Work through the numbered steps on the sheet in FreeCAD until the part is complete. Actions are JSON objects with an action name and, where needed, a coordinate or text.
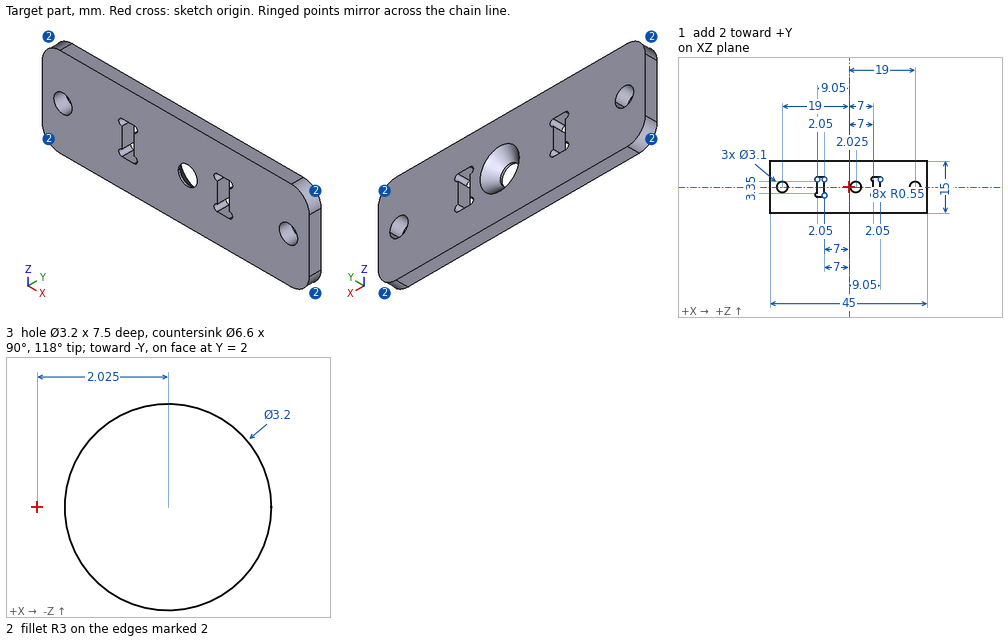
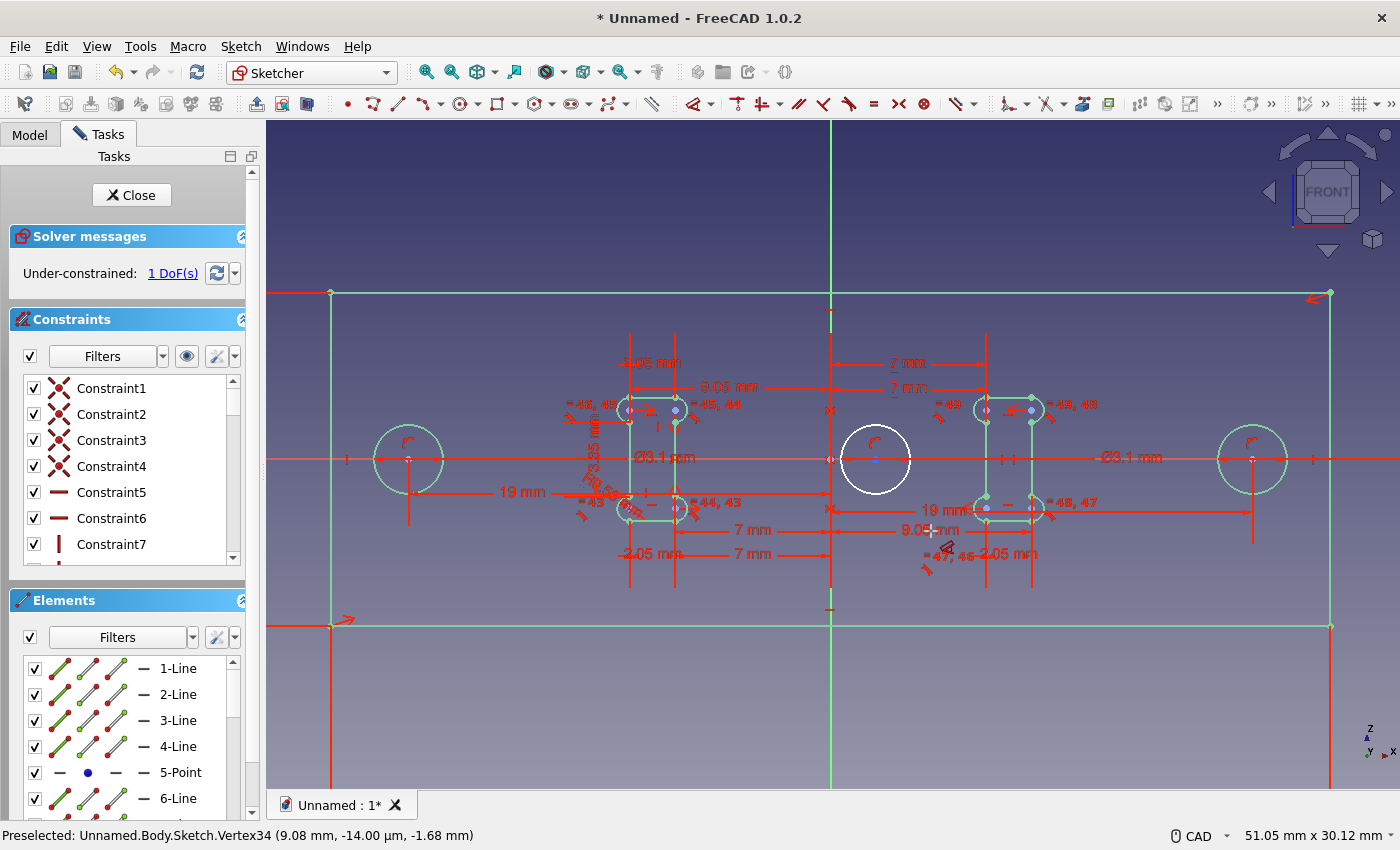
{"action": "left_click", "coordinate": [876, 459]}
{"action": "left_click", "coordinate": [853, 517]}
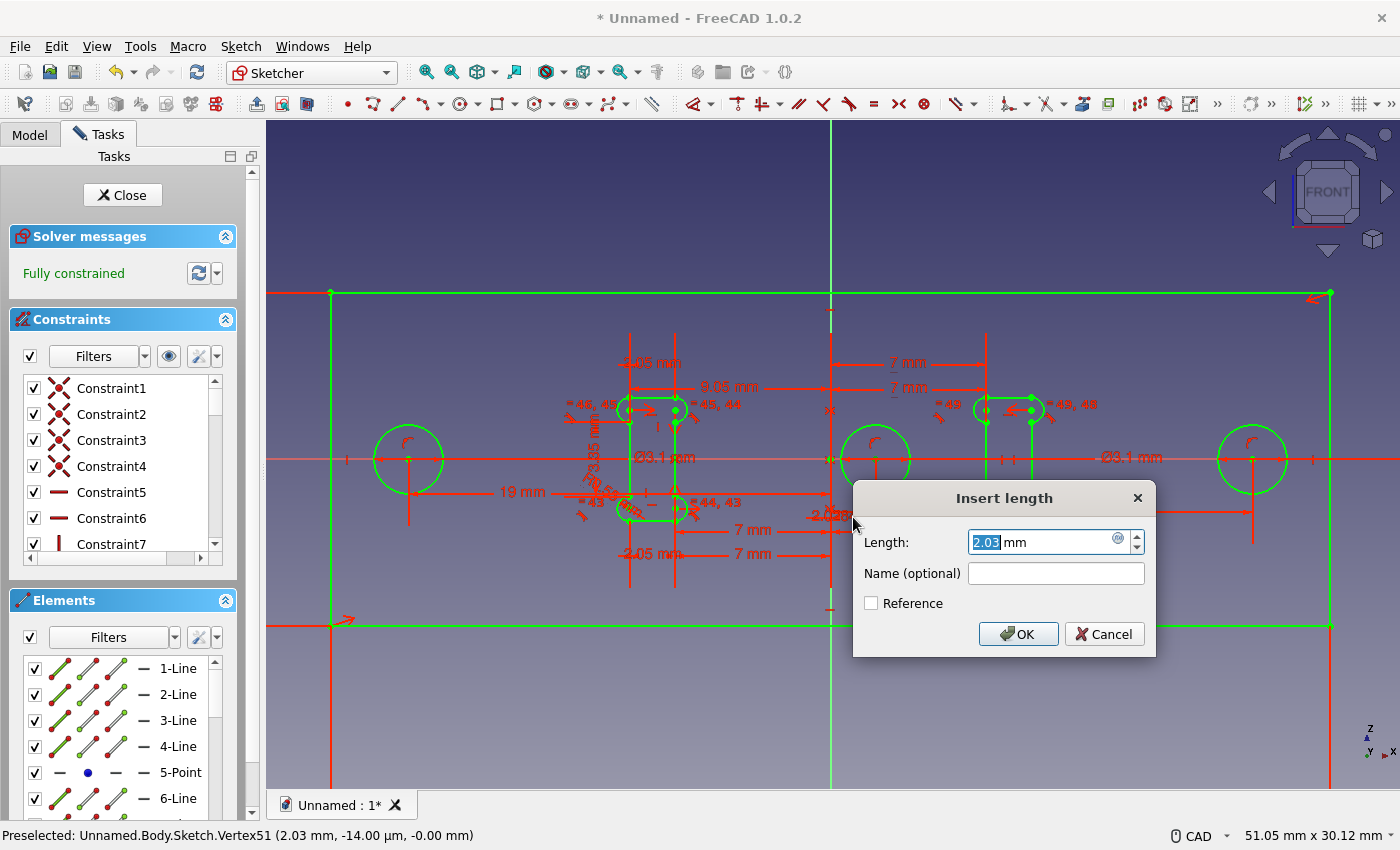
{"action": "type", "text": "2.025"}
{"action": "key", "text": "Return"}
{"action": "key", "text": "Escape"}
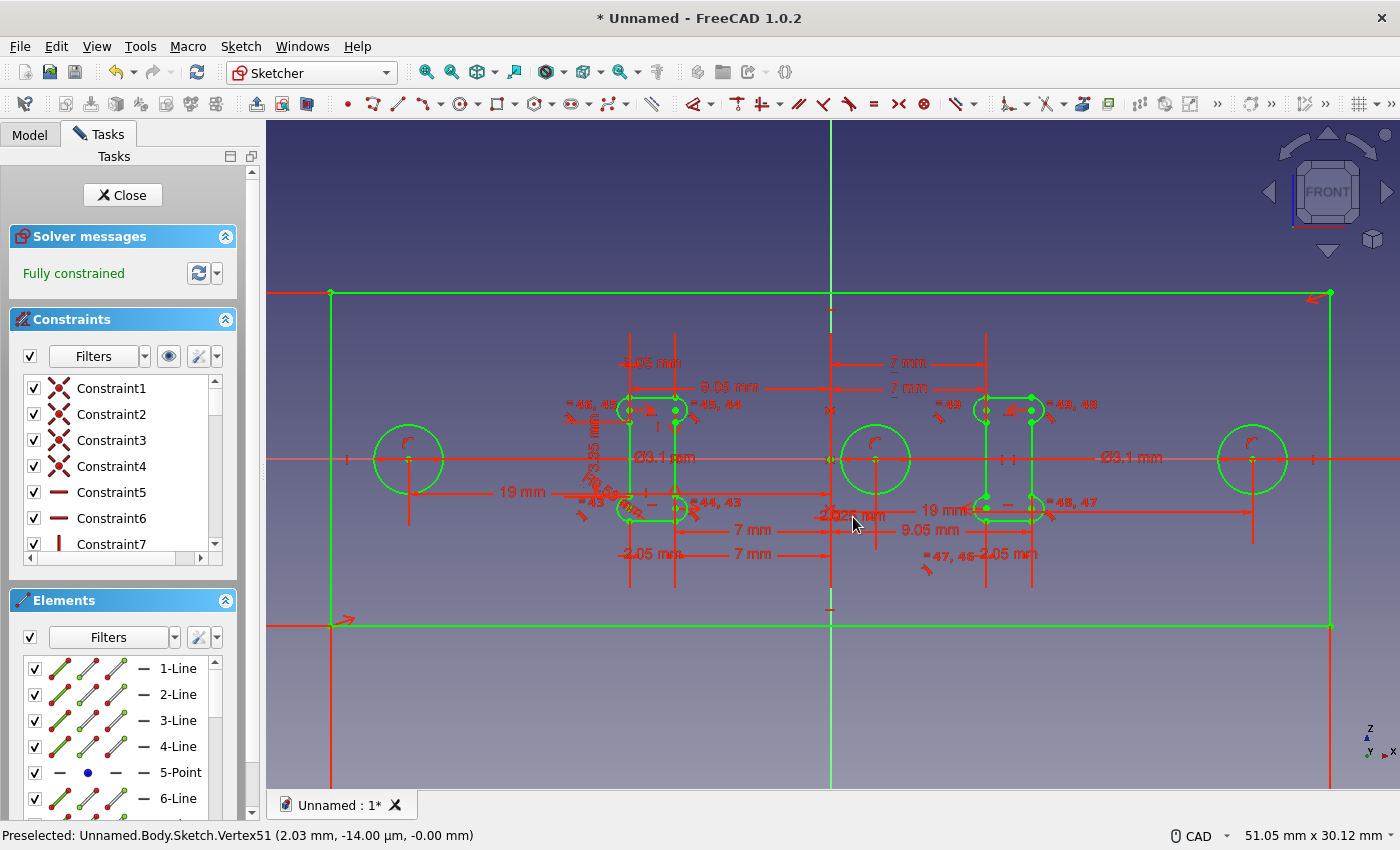
{"action": "left_click", "coordinate": [123, 195]}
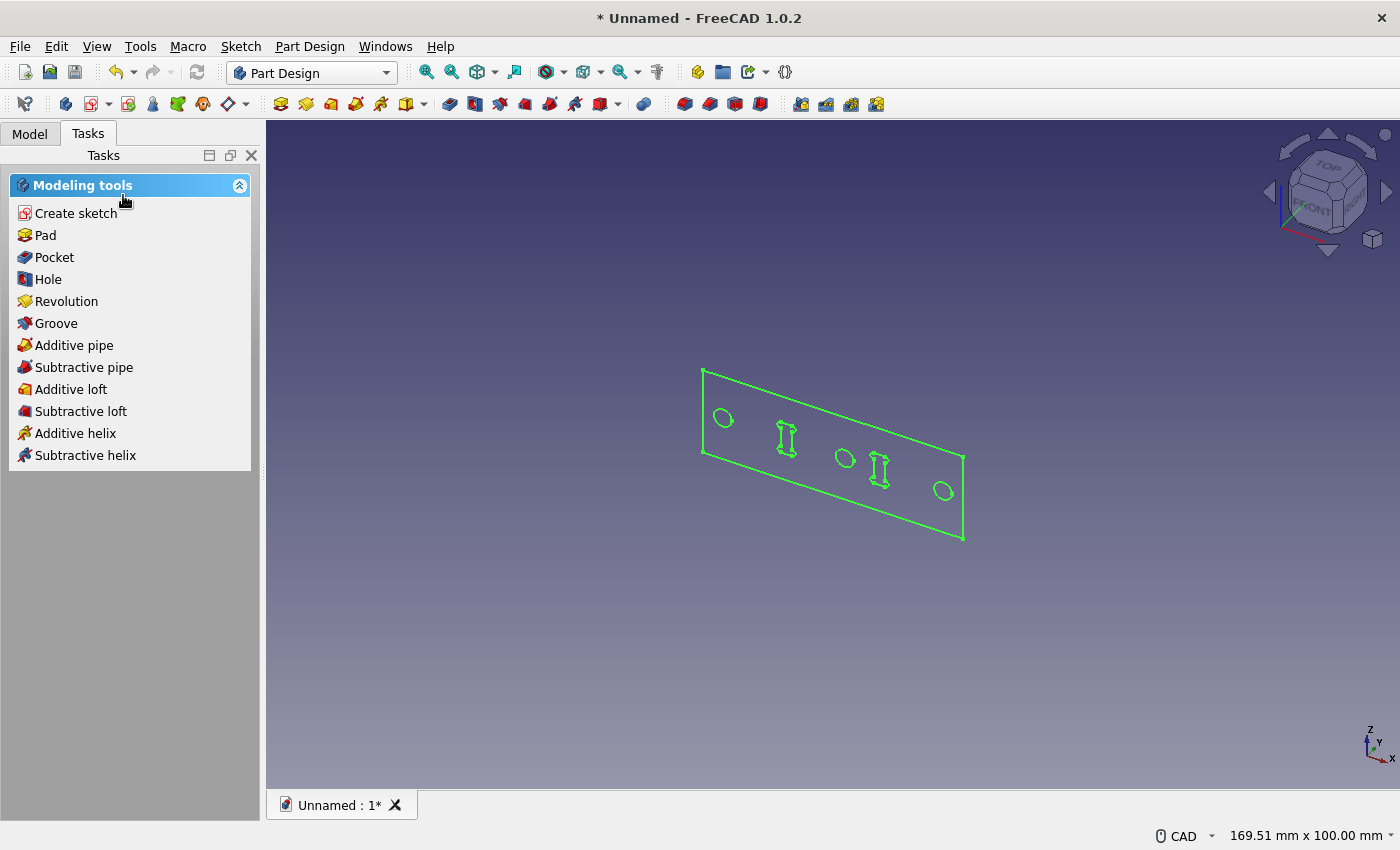
{"action": "left_click", "coordinate": [281, 104]}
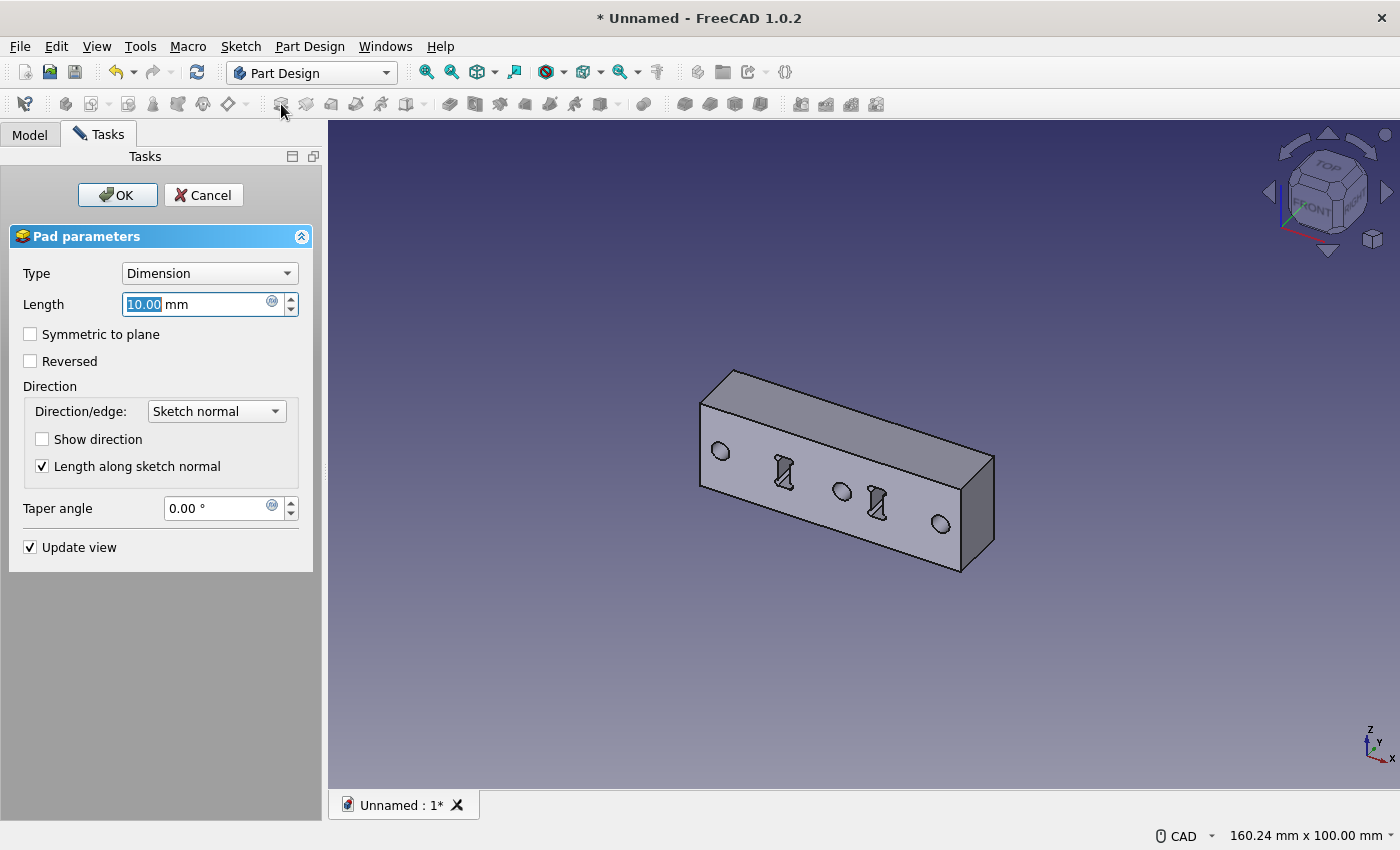
{"action": "type", "text": "2"}
{"action": "key", "text": "Tab"}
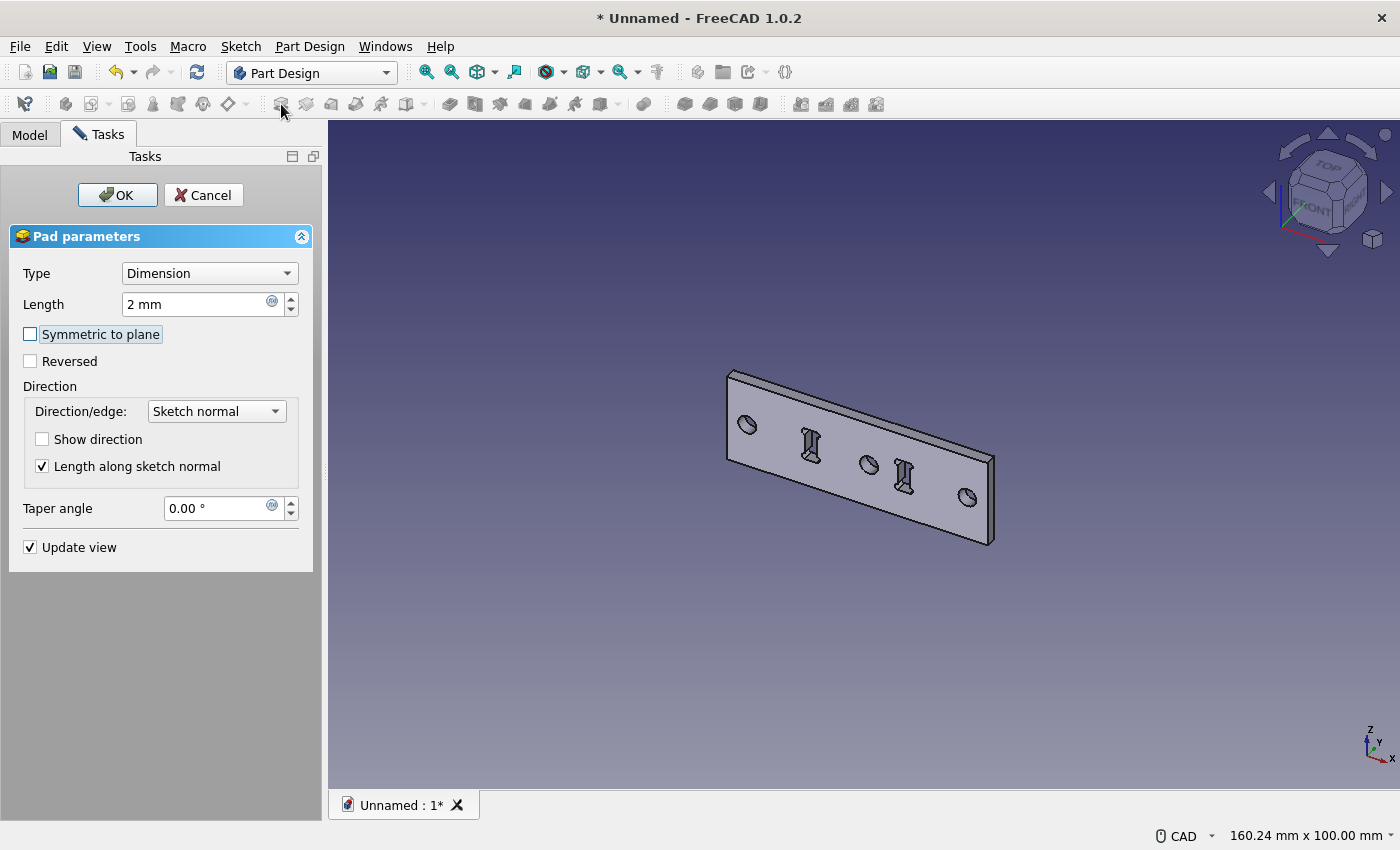
{"action": "left_click", "coordinate": [31, 361]}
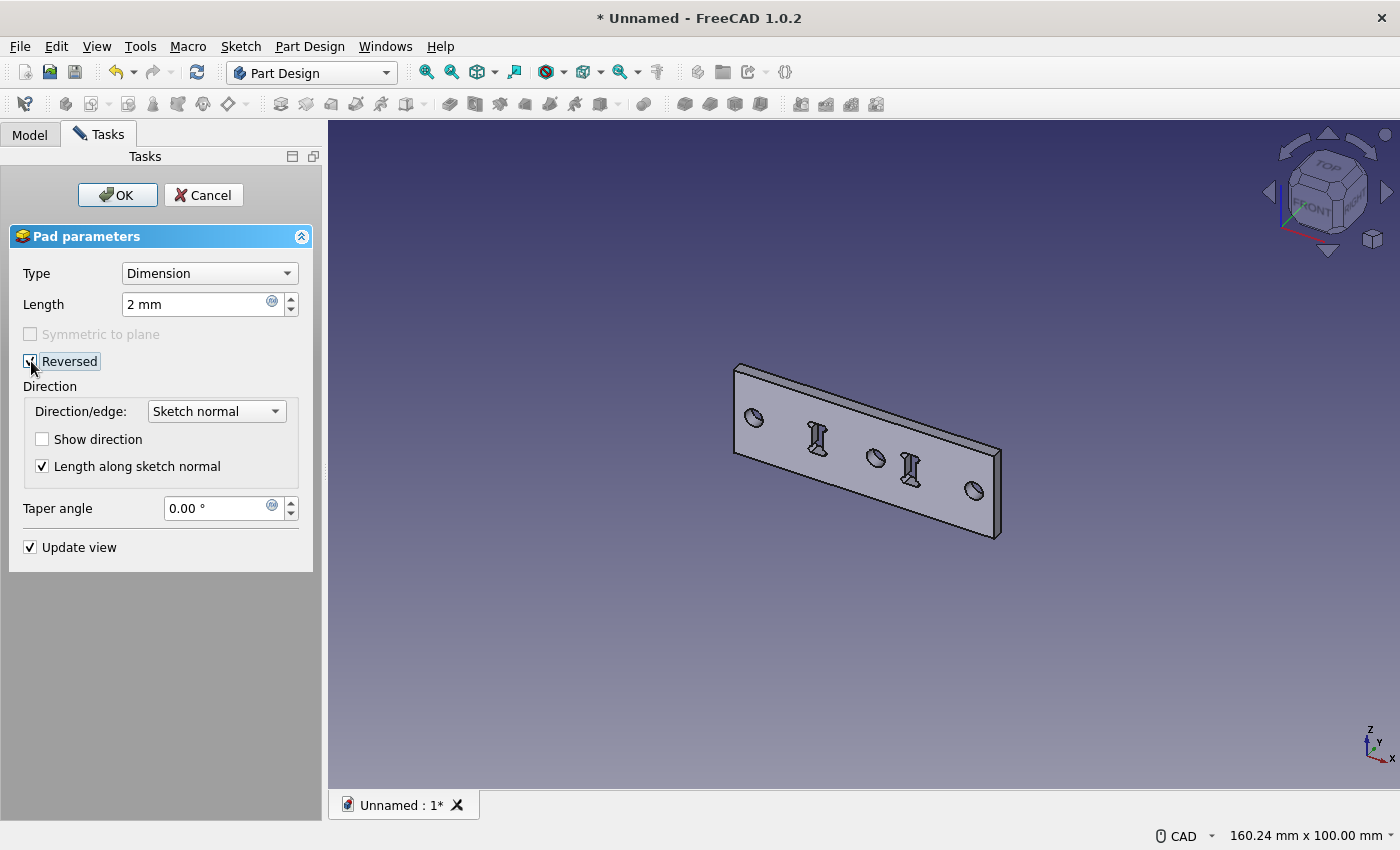
{"action": "left_click", "coordinate": [118, 195]}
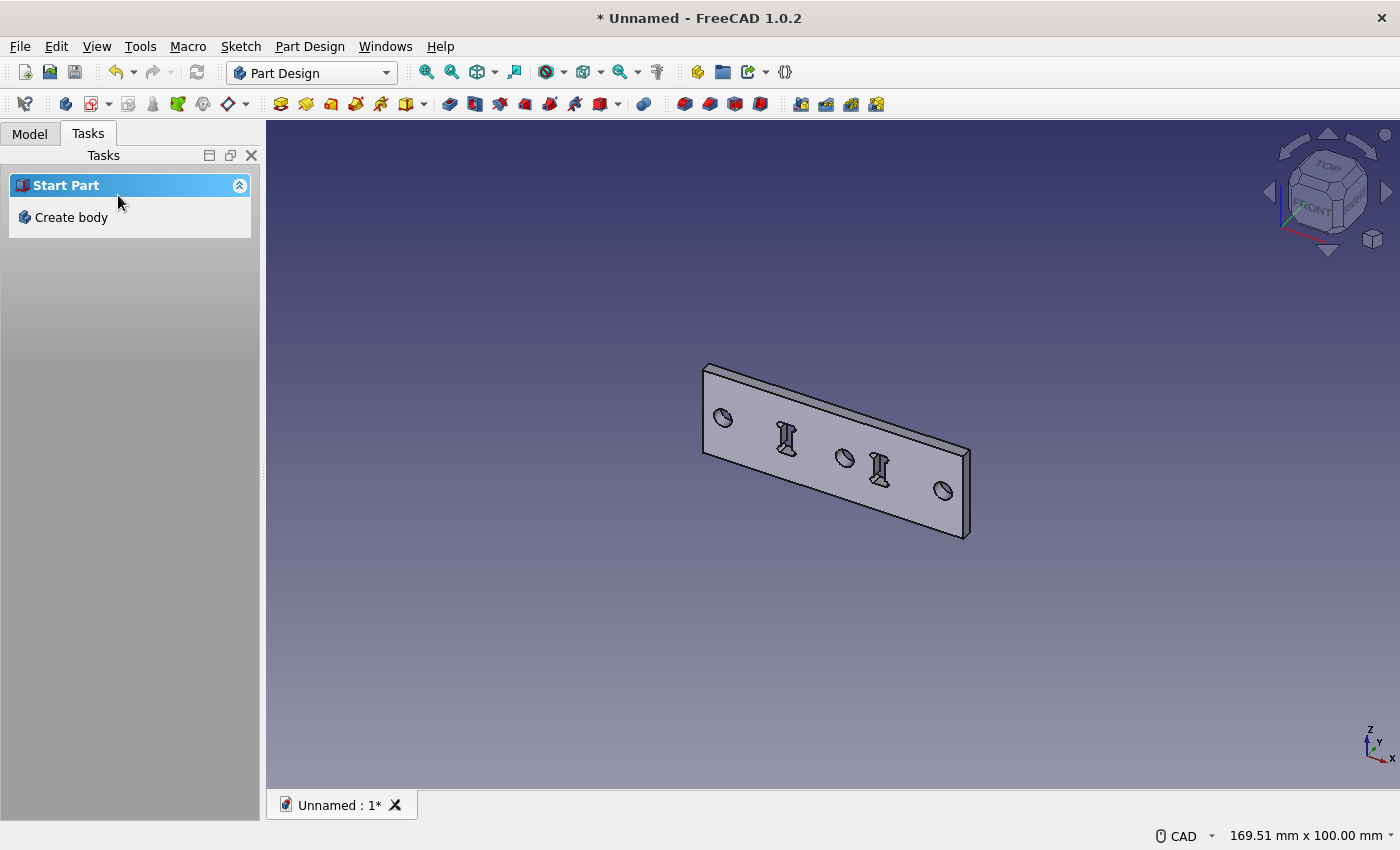
{"action": "left_click", "coordinate": [427, 72]}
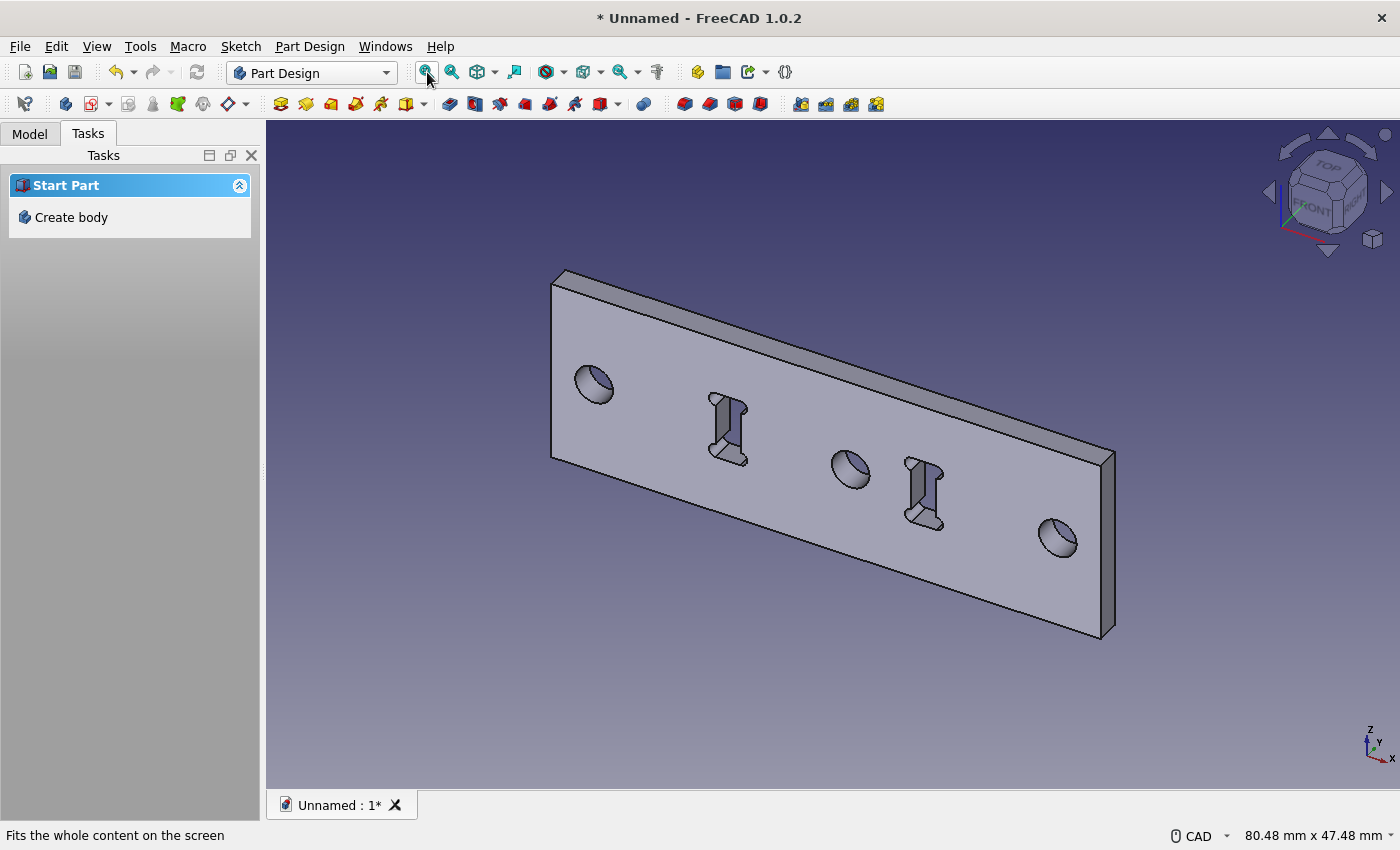
{"action": "left_click", "coordinate": [1108, 458]}